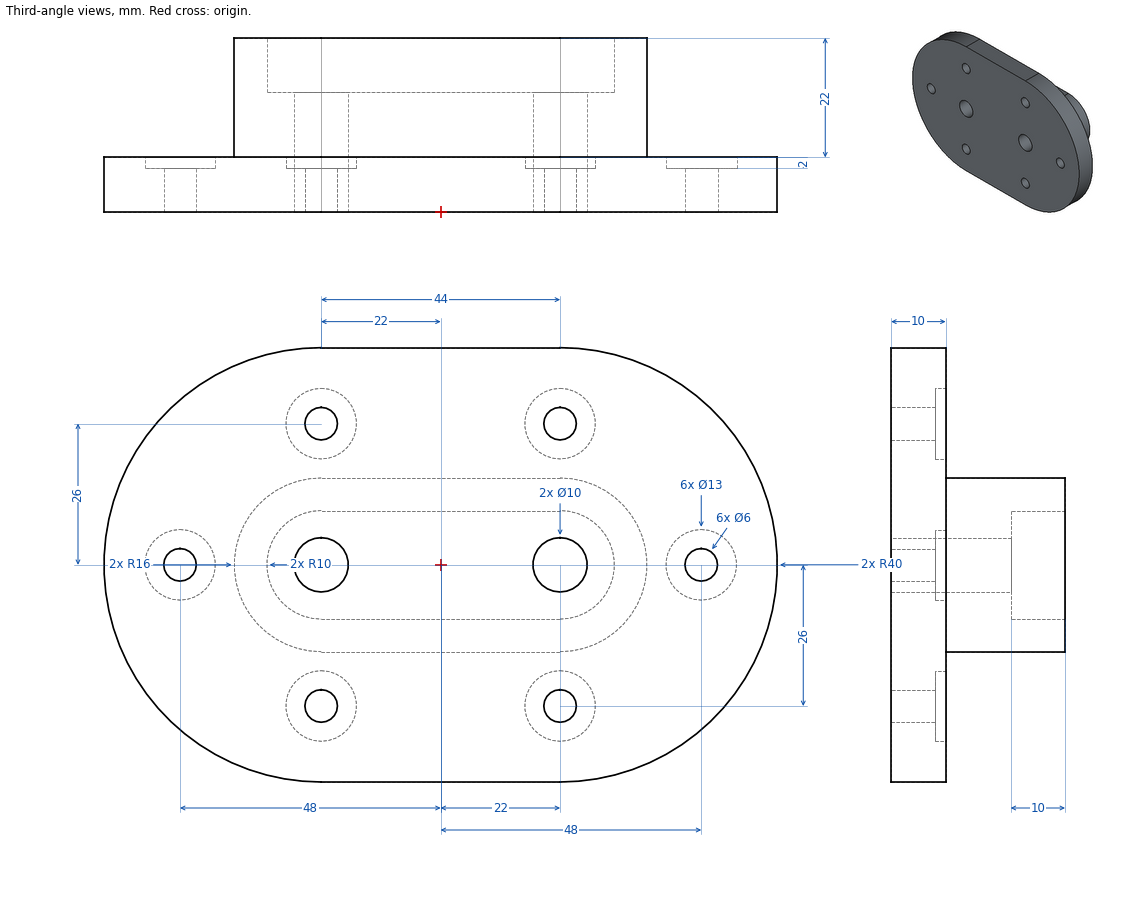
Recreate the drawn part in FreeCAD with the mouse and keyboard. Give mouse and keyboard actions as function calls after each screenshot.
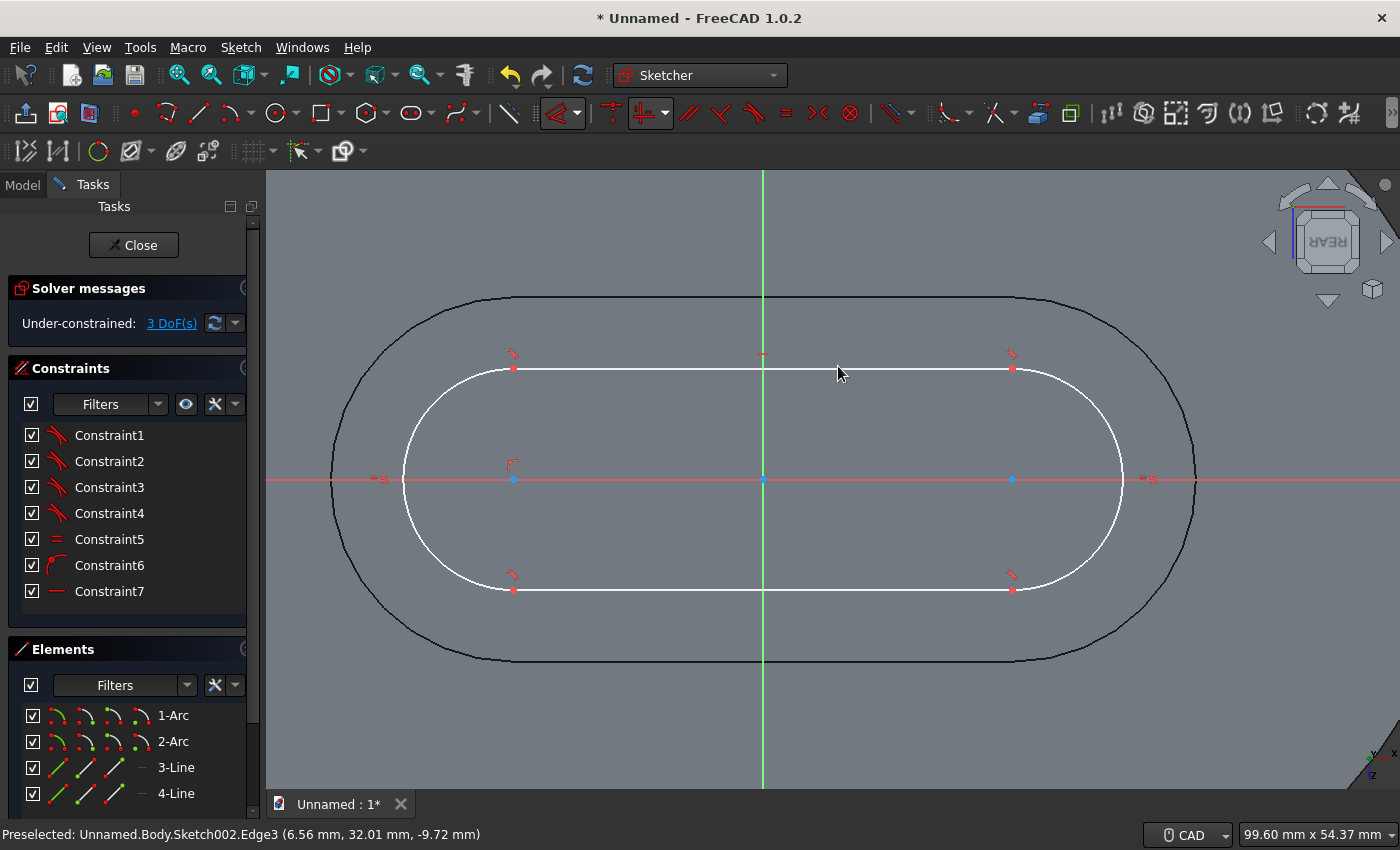
click(425, 414)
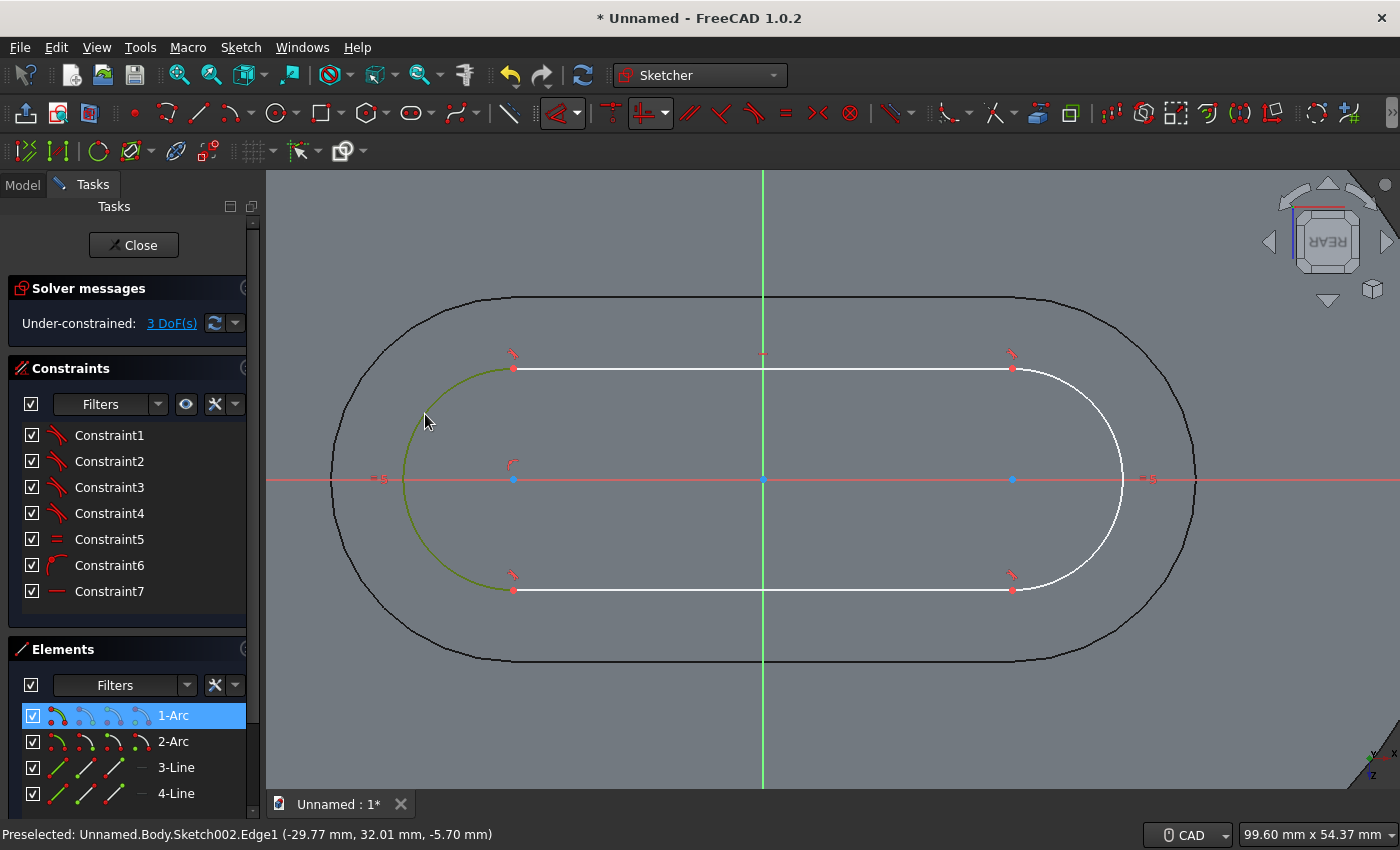
click(580, 114)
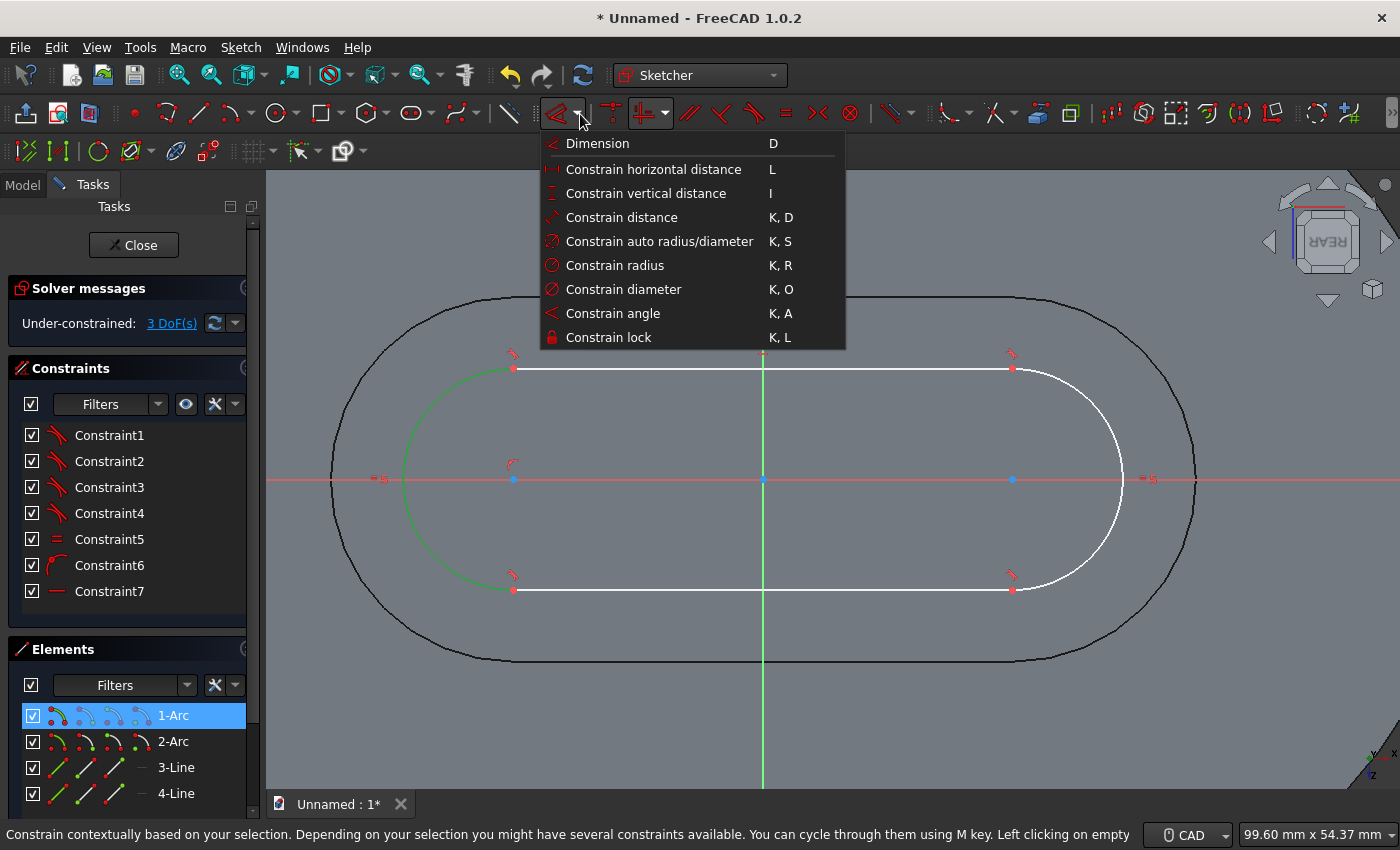
click(693, 265)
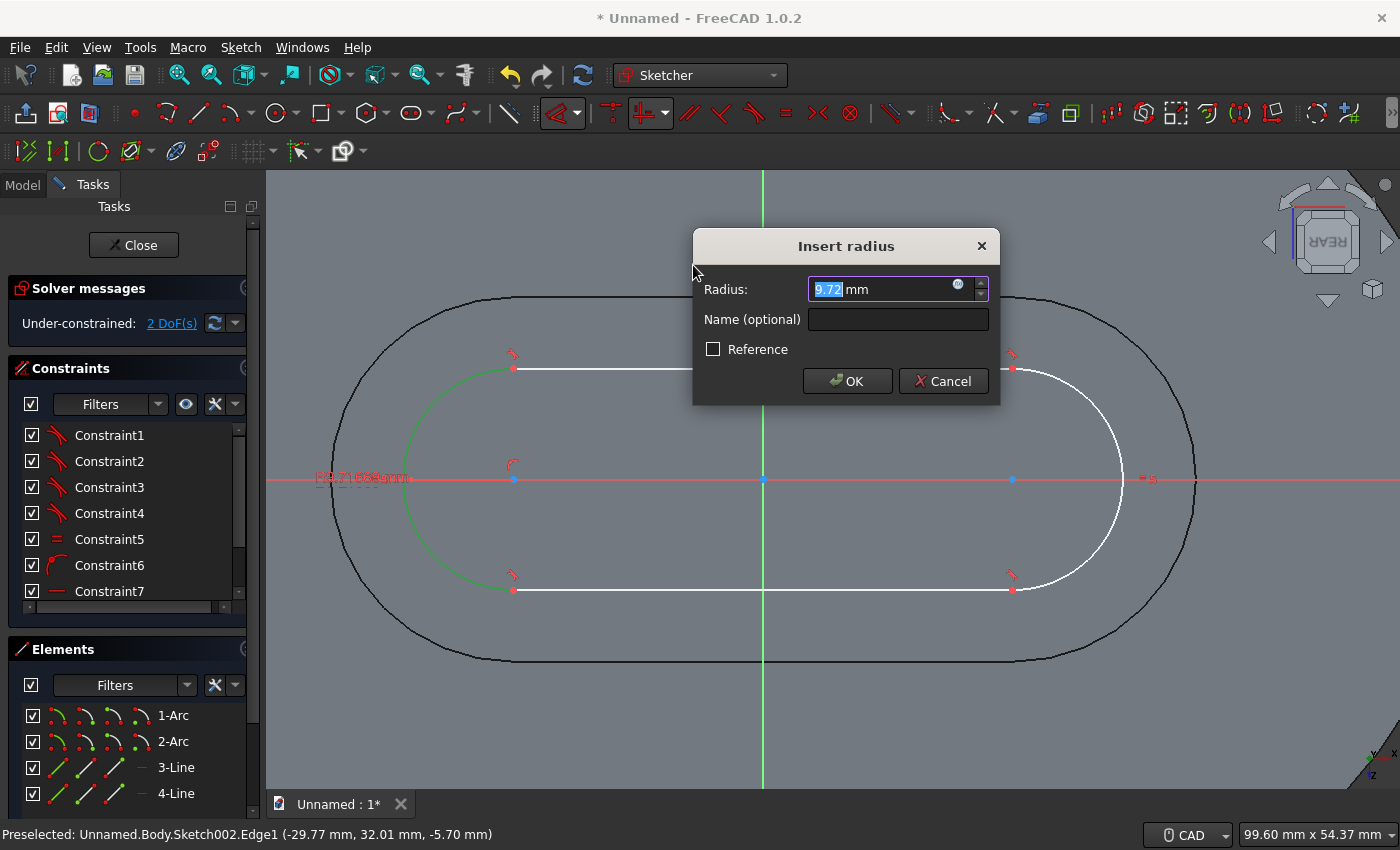
text(10)
key(Return)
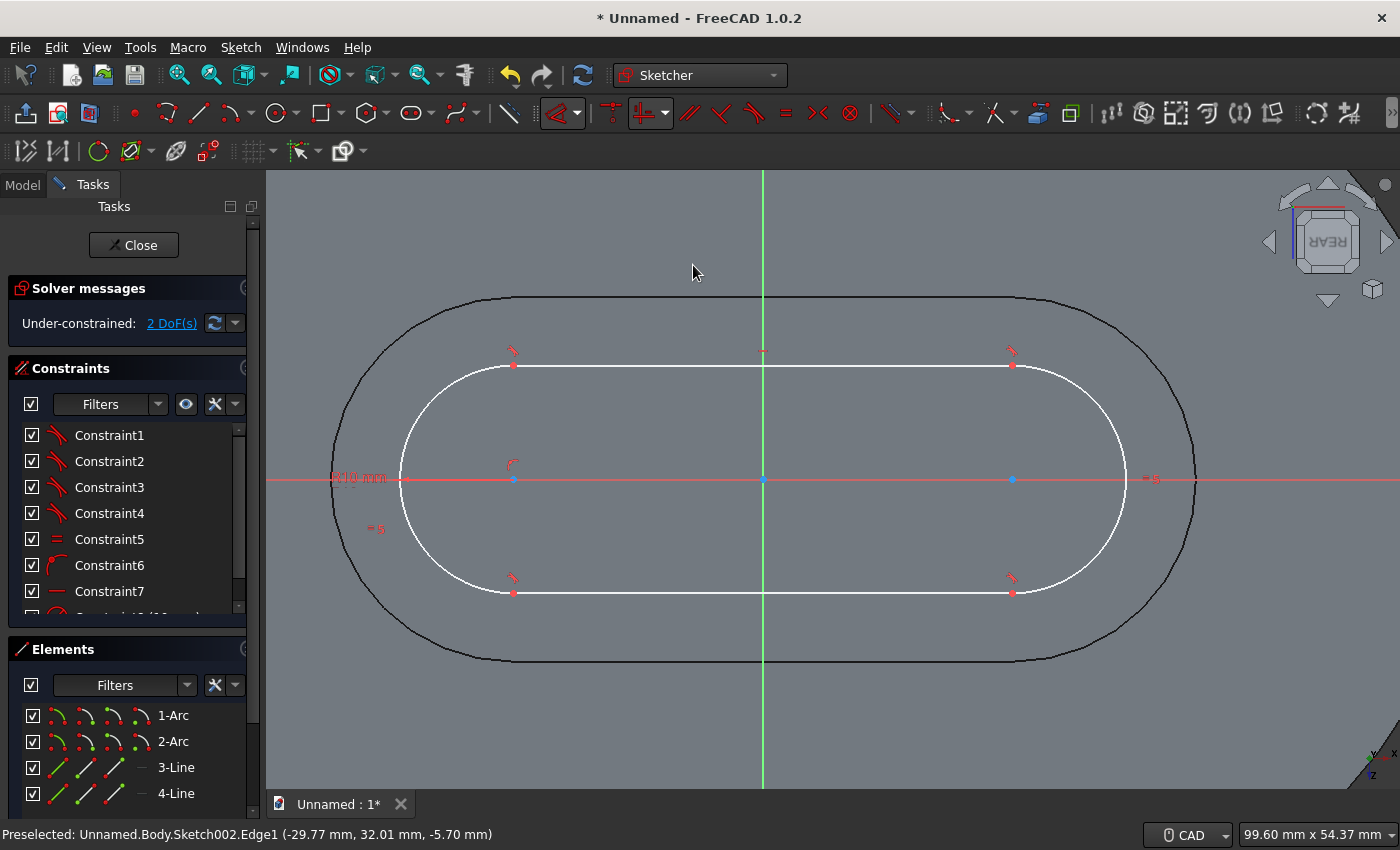
click(663, 366)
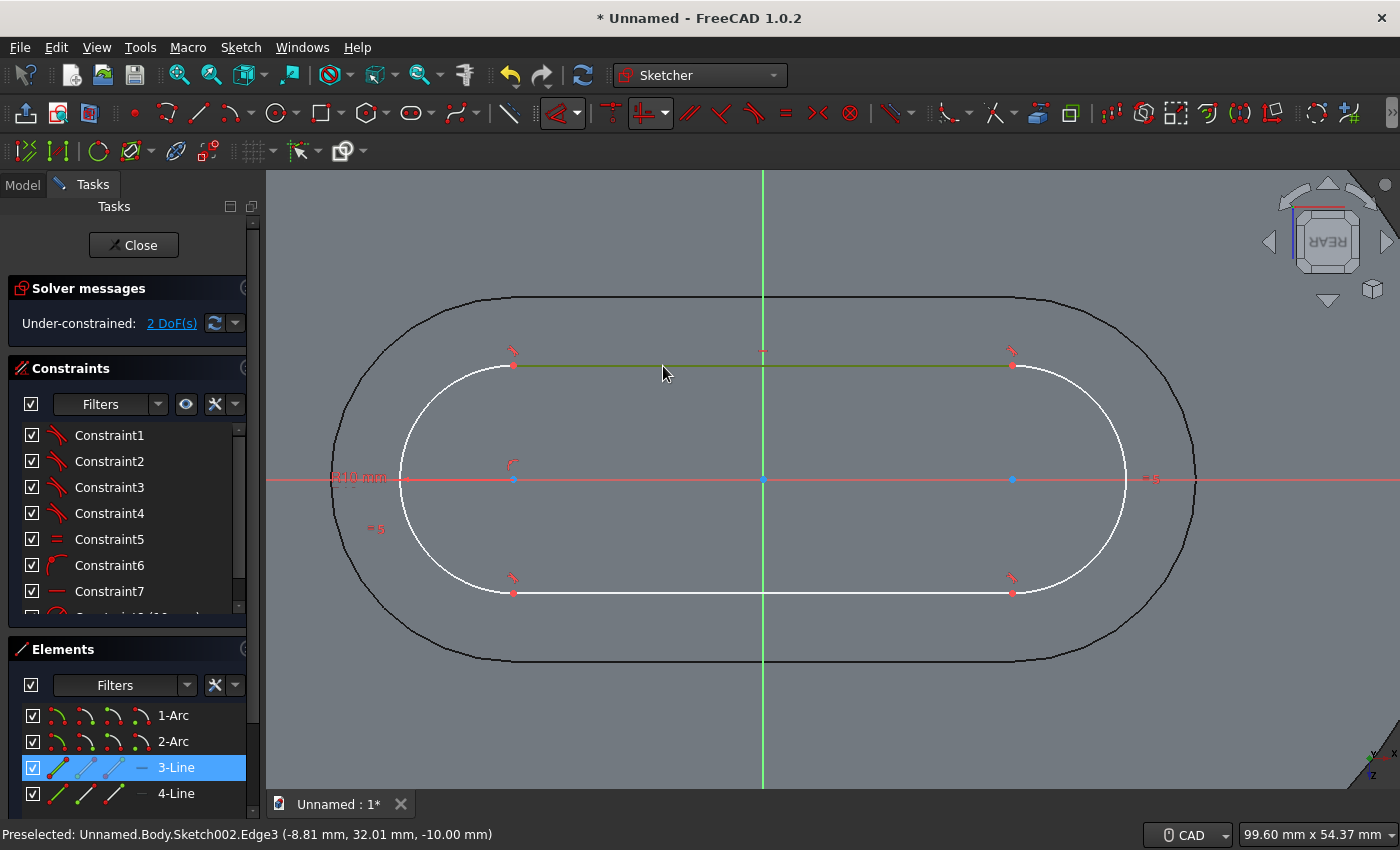
key(l)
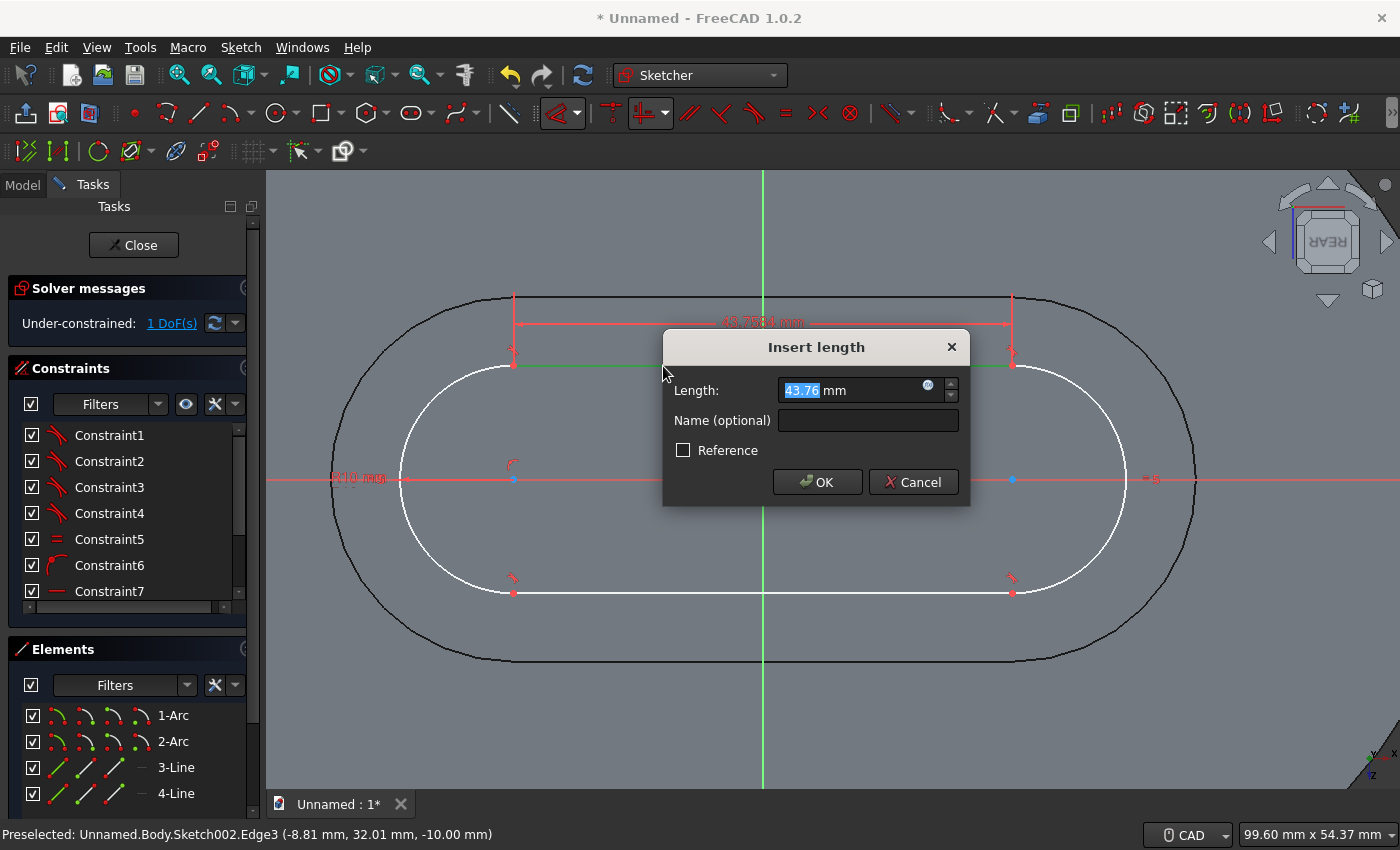
text(44)
key(Return)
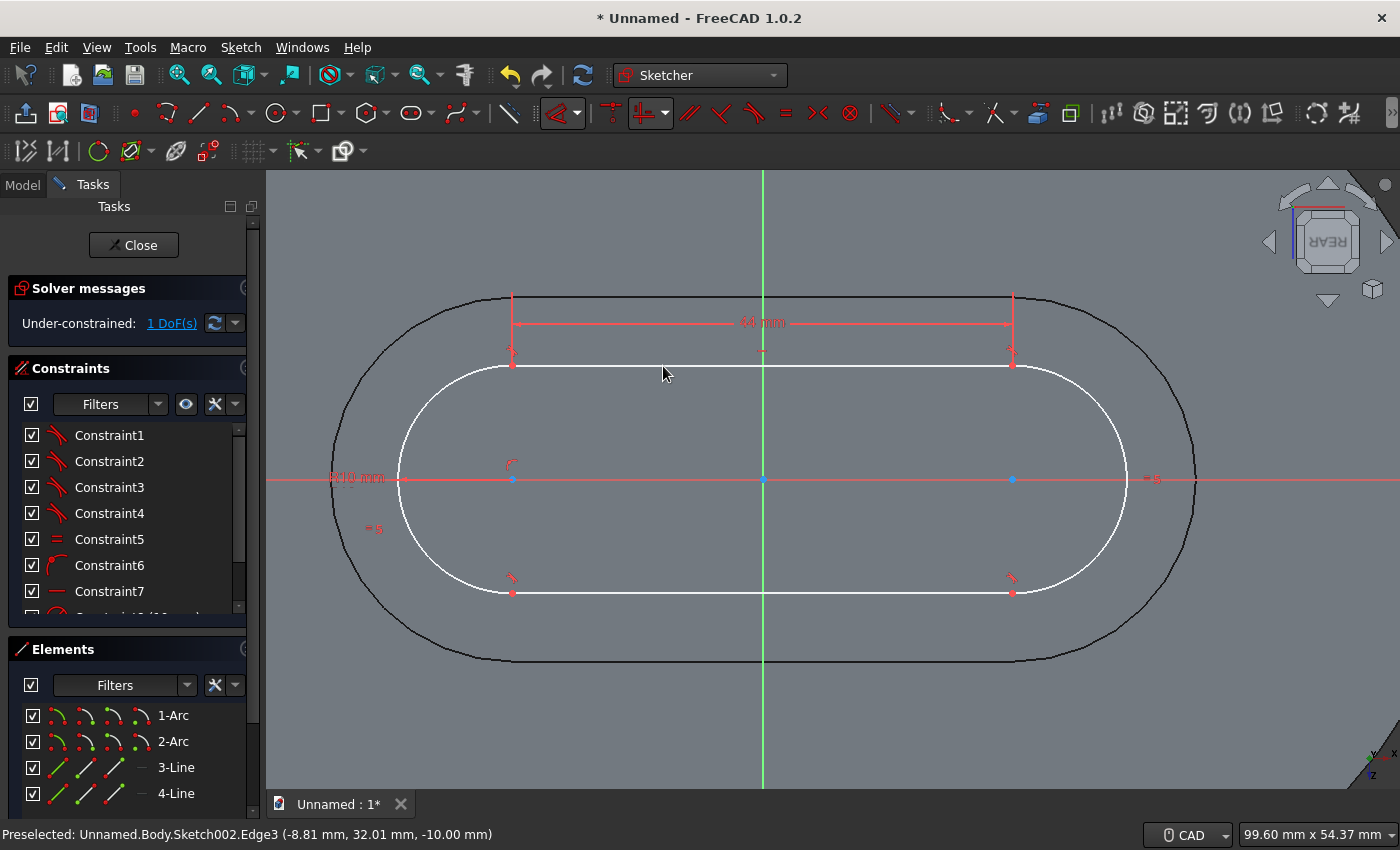
click(512, 366)